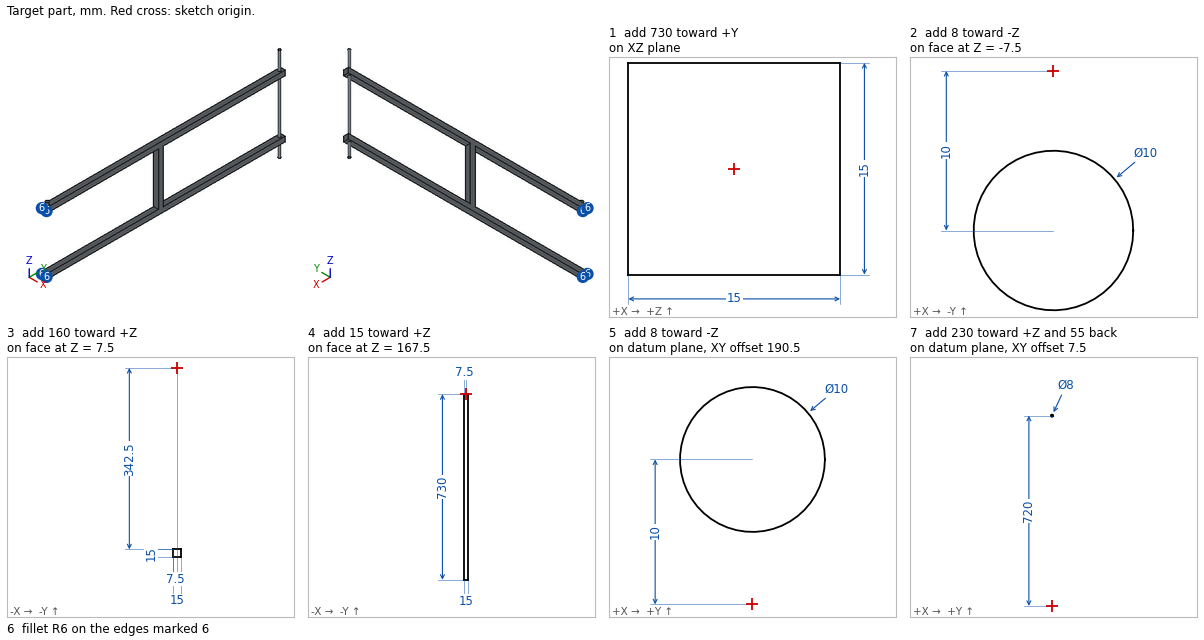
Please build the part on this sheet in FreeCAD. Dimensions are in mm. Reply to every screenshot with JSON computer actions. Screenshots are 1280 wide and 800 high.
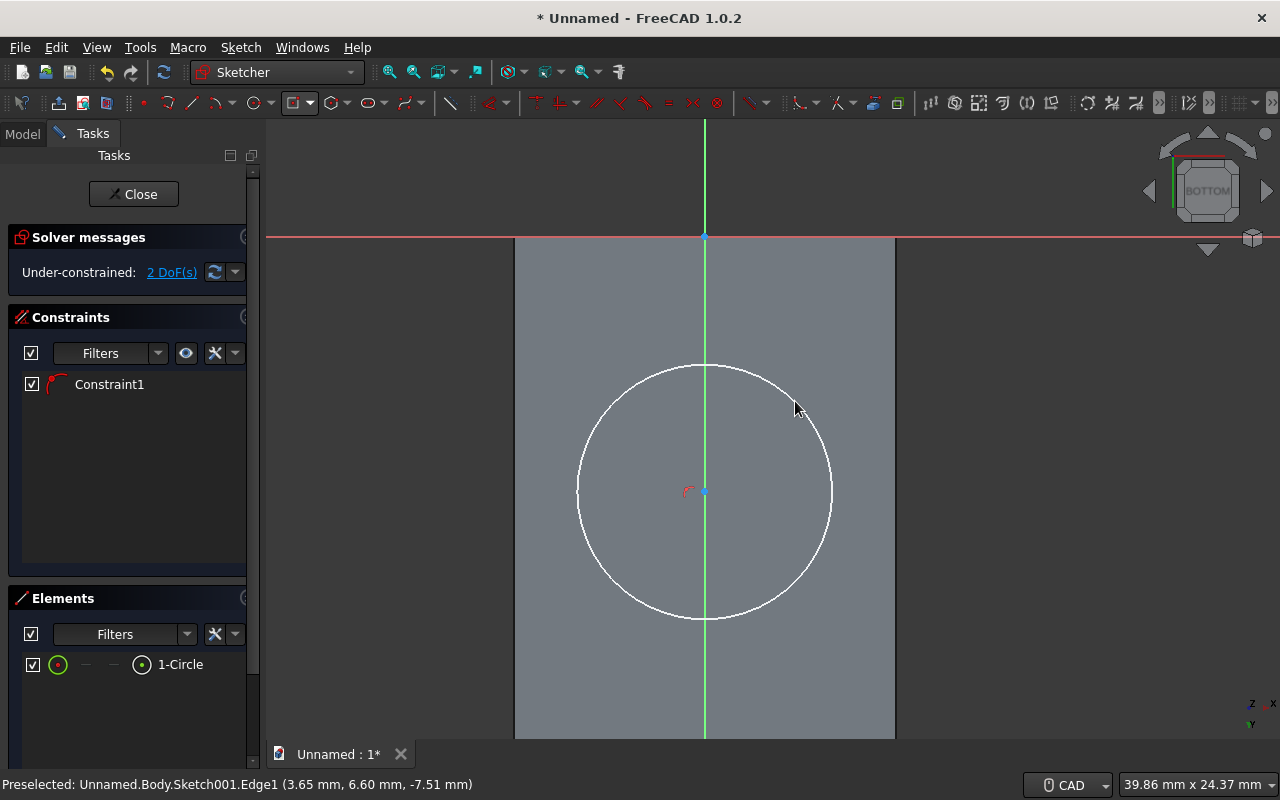
{"action": "left_click", "coordinate": [490, 104]}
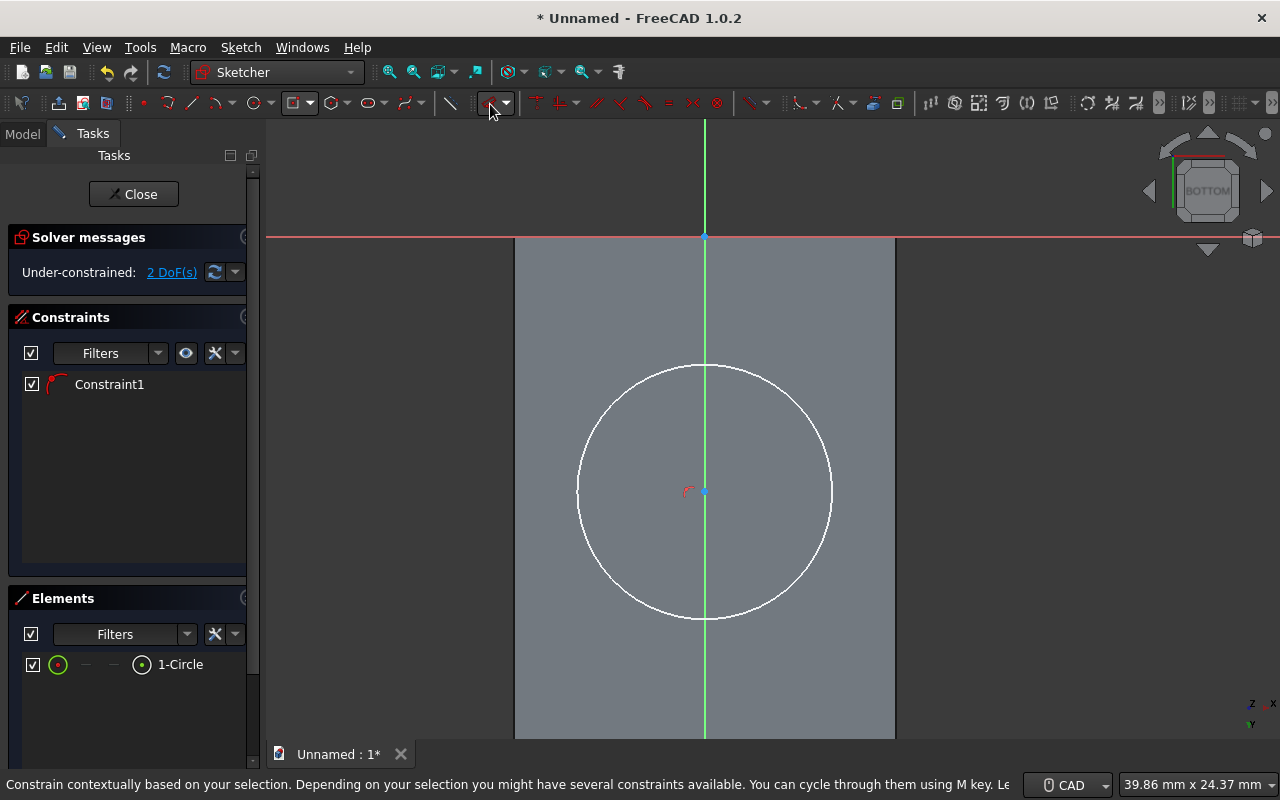
{"action": "left_click", "coordinate": [795, 402]}
{"action": "left_click", "coordinate": [818, 379]}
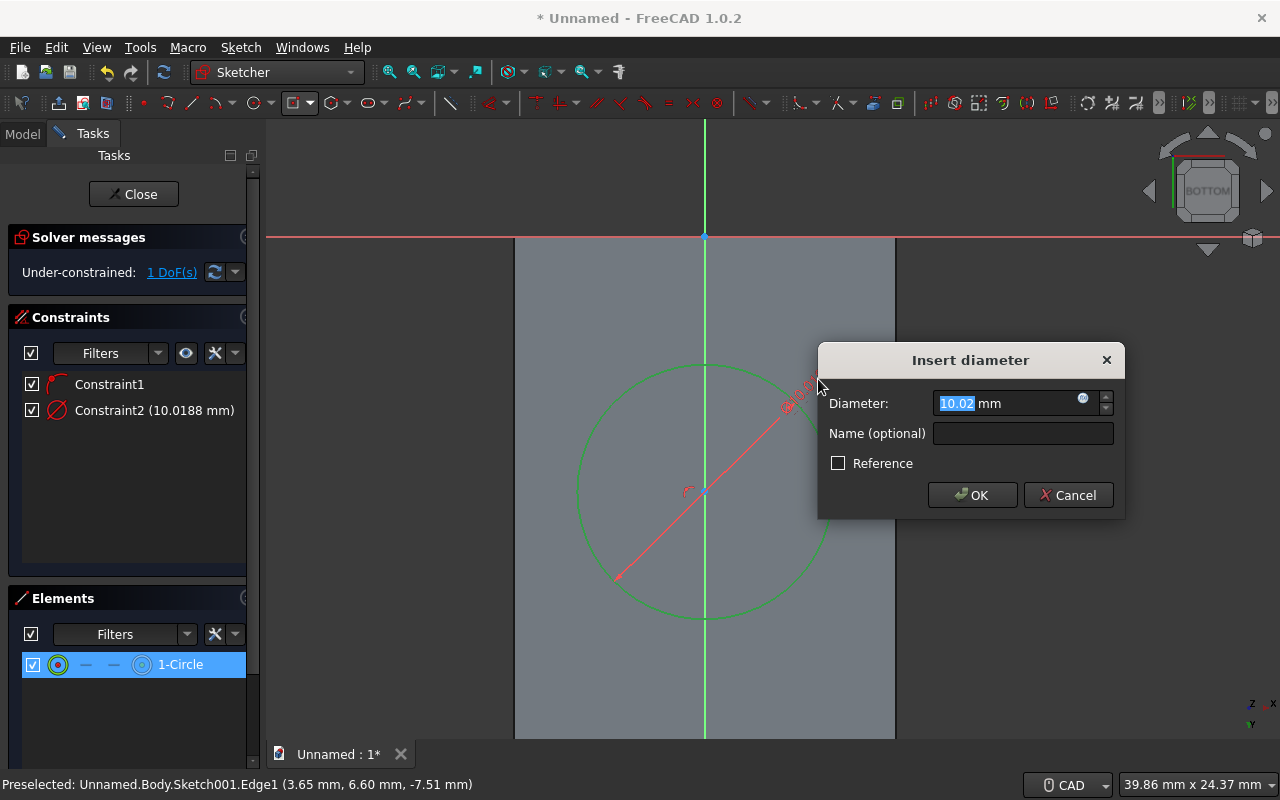
{"action": "type", "text": "10"}
{"action": "key", "text": "Return"}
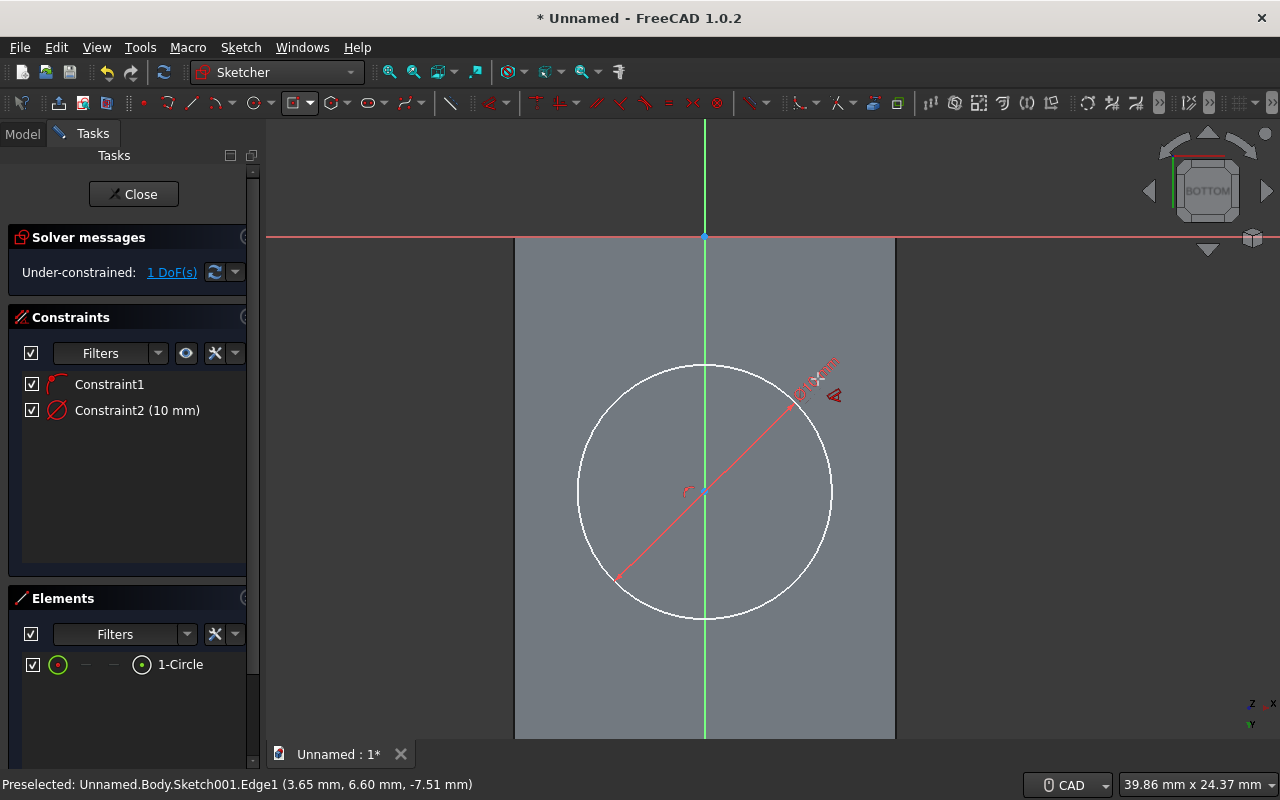
{"action": "left_click", "coordinate": [705, 492]}
{"action": "left_click", "coordinate": [739, 306]}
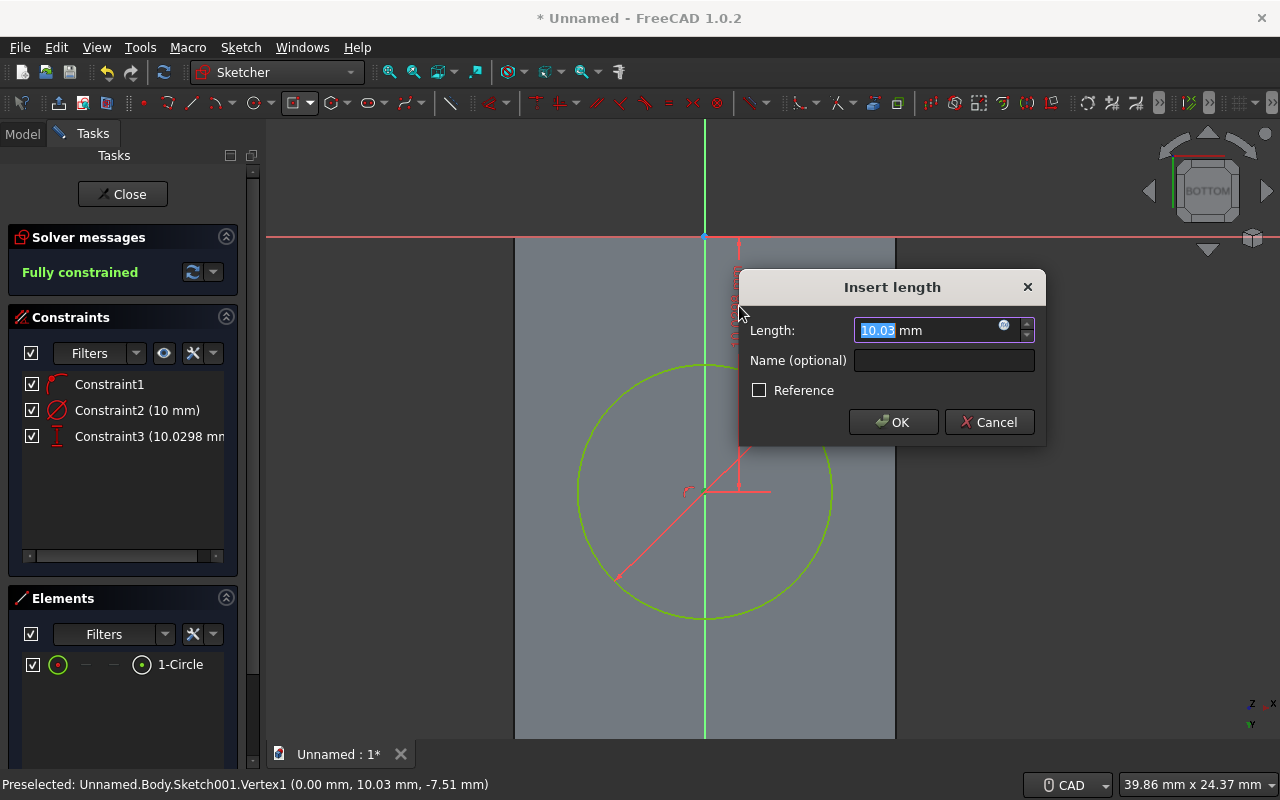
{"action": "type", "text": "10"}
{"action": "key", "text": "Return"}
{"action": "key", "text": "Escape"}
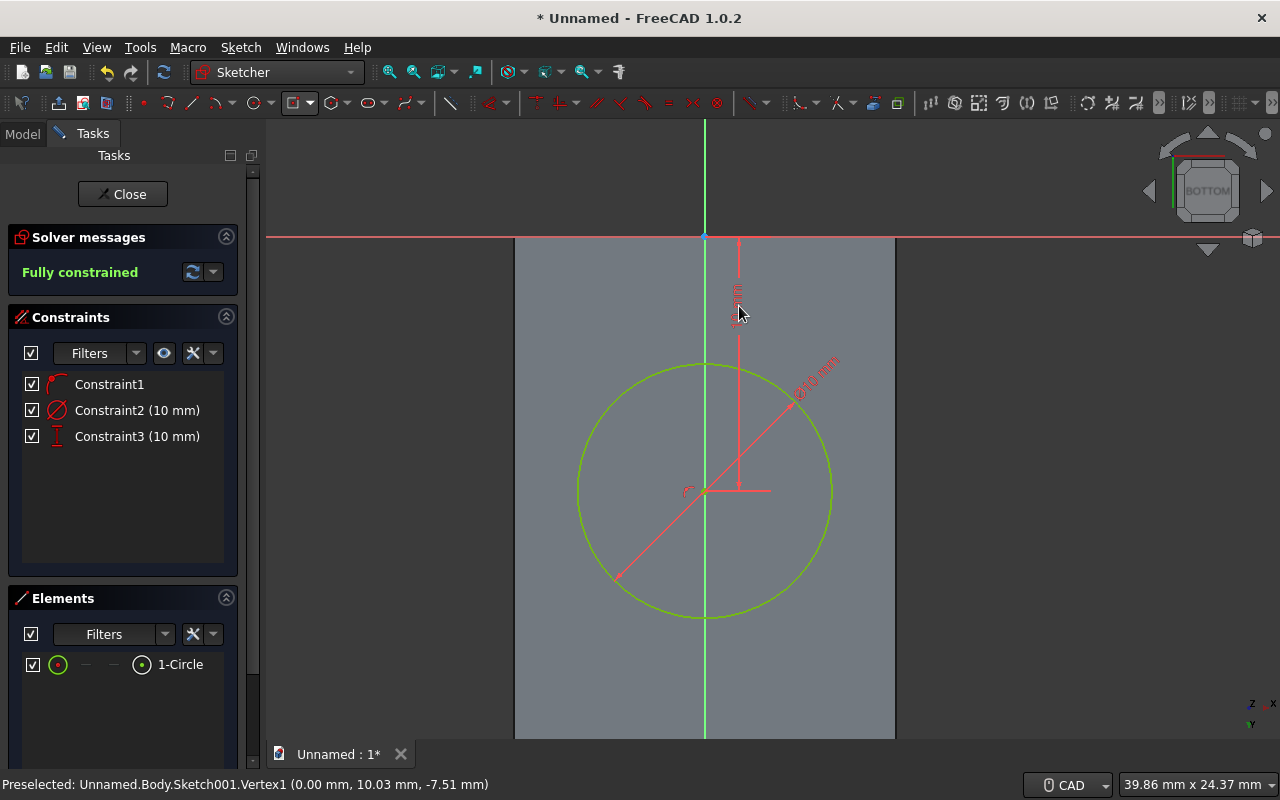
{"action": "left_click", "coordinate": [123, 194]}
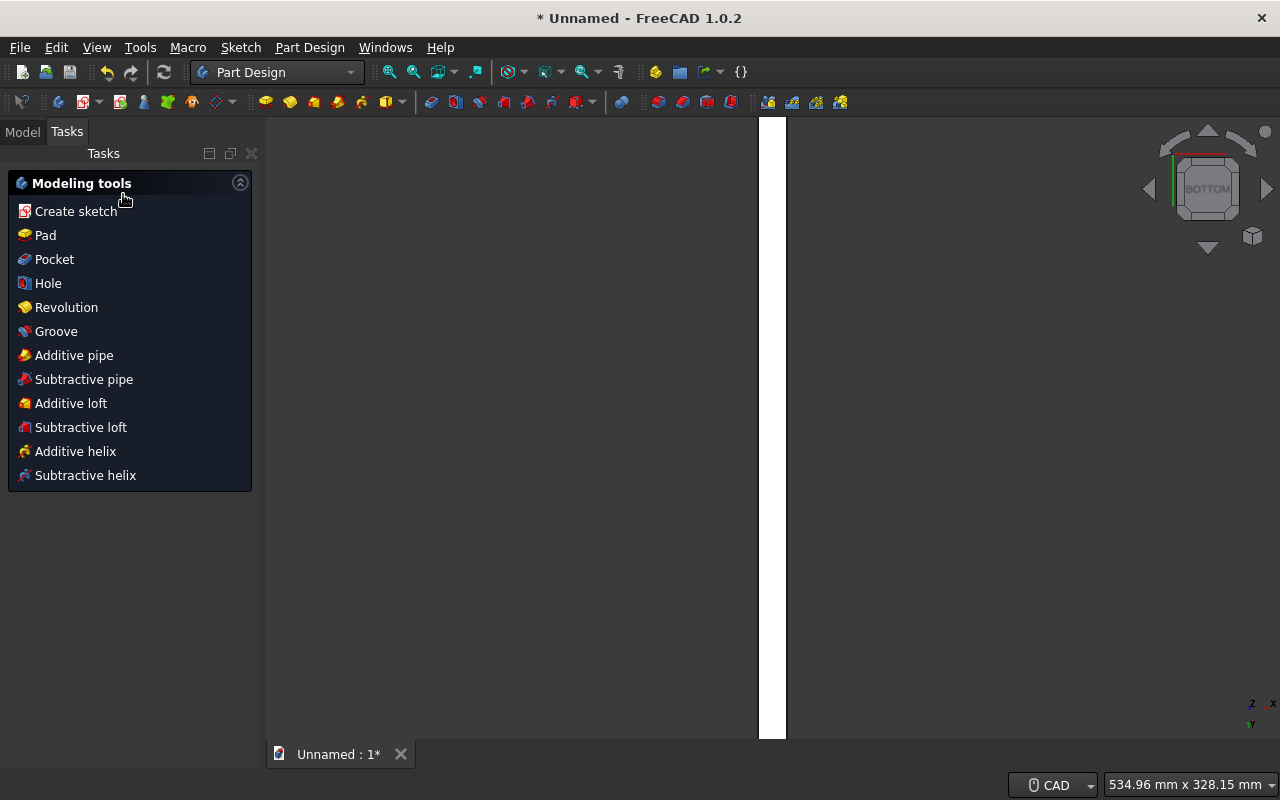
{"action": "left_click", "coordinate": [266, 102]}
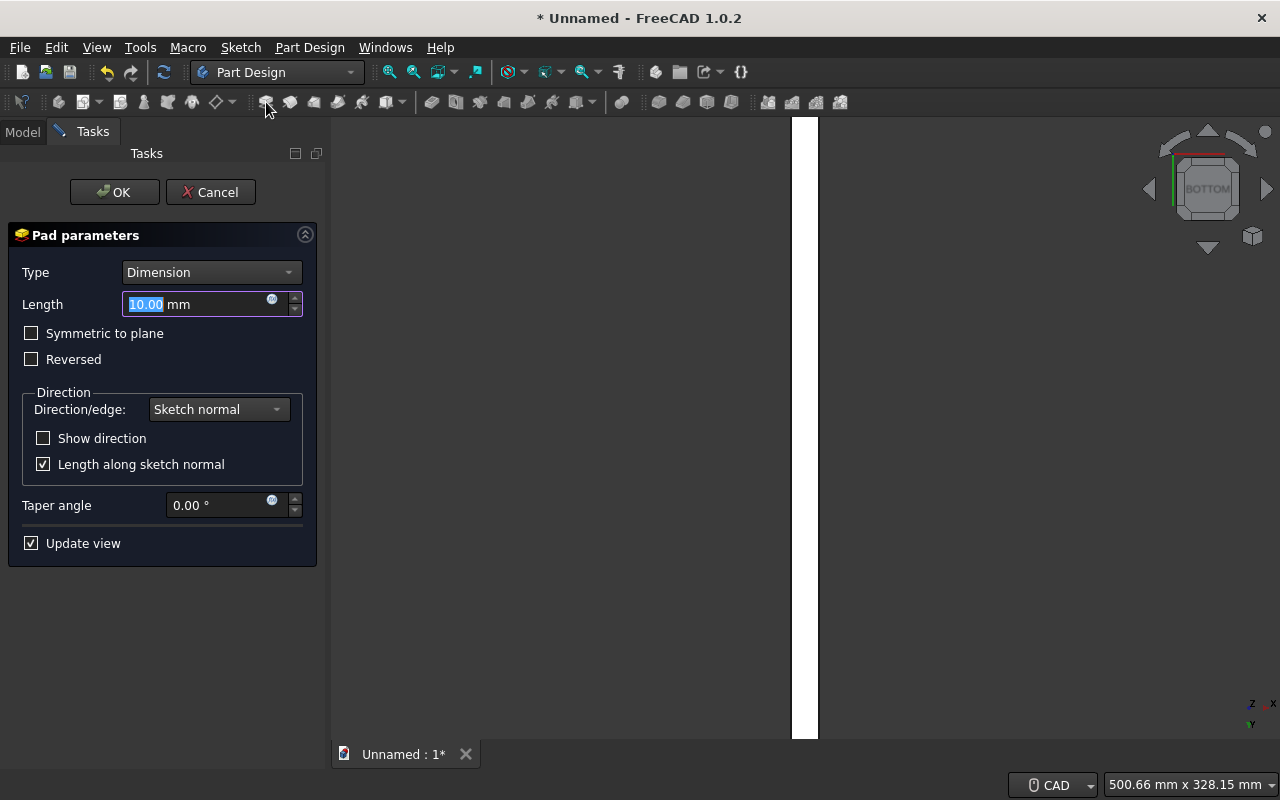
{"action": "type", "text": "8"}
{"action": "key", "text": "Tab"}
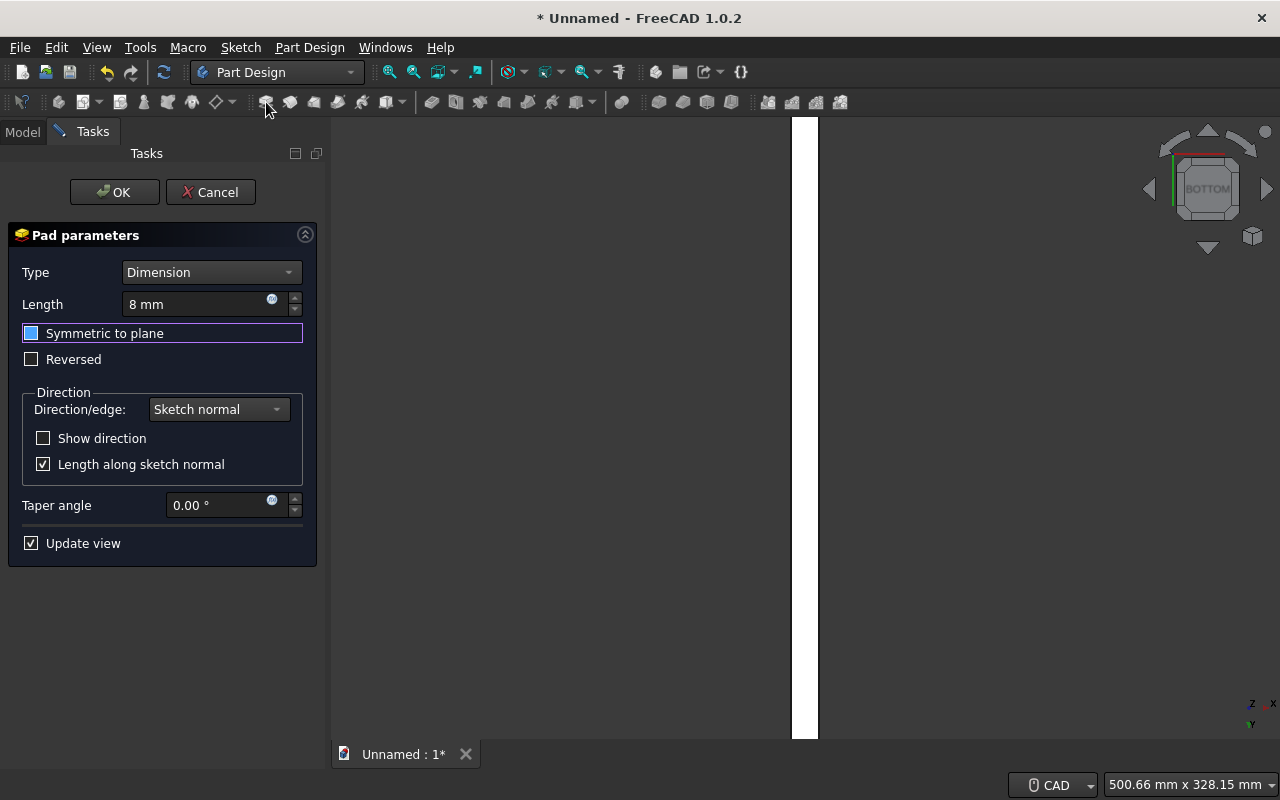
{"action": "left_click", "coordinate": [115, 192]}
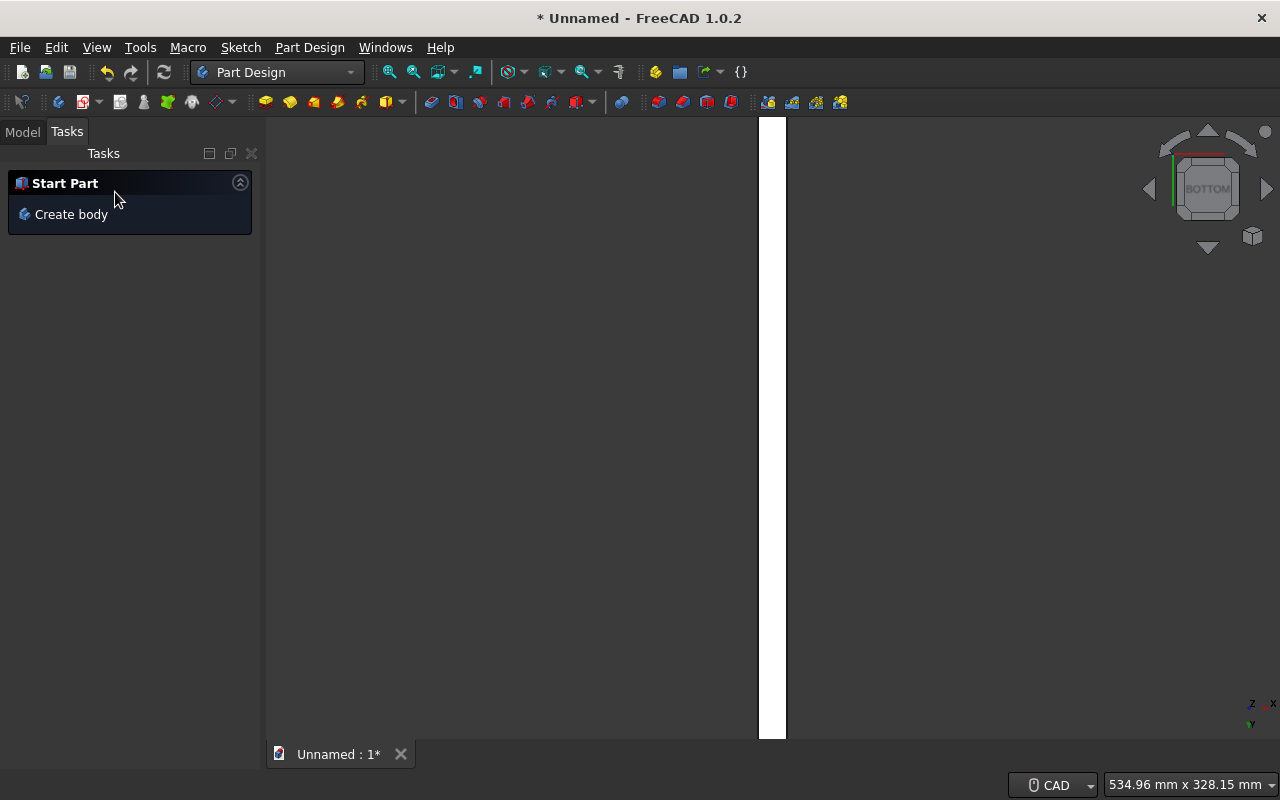
{"action": "left_click", "coordinate": [390, 72]}